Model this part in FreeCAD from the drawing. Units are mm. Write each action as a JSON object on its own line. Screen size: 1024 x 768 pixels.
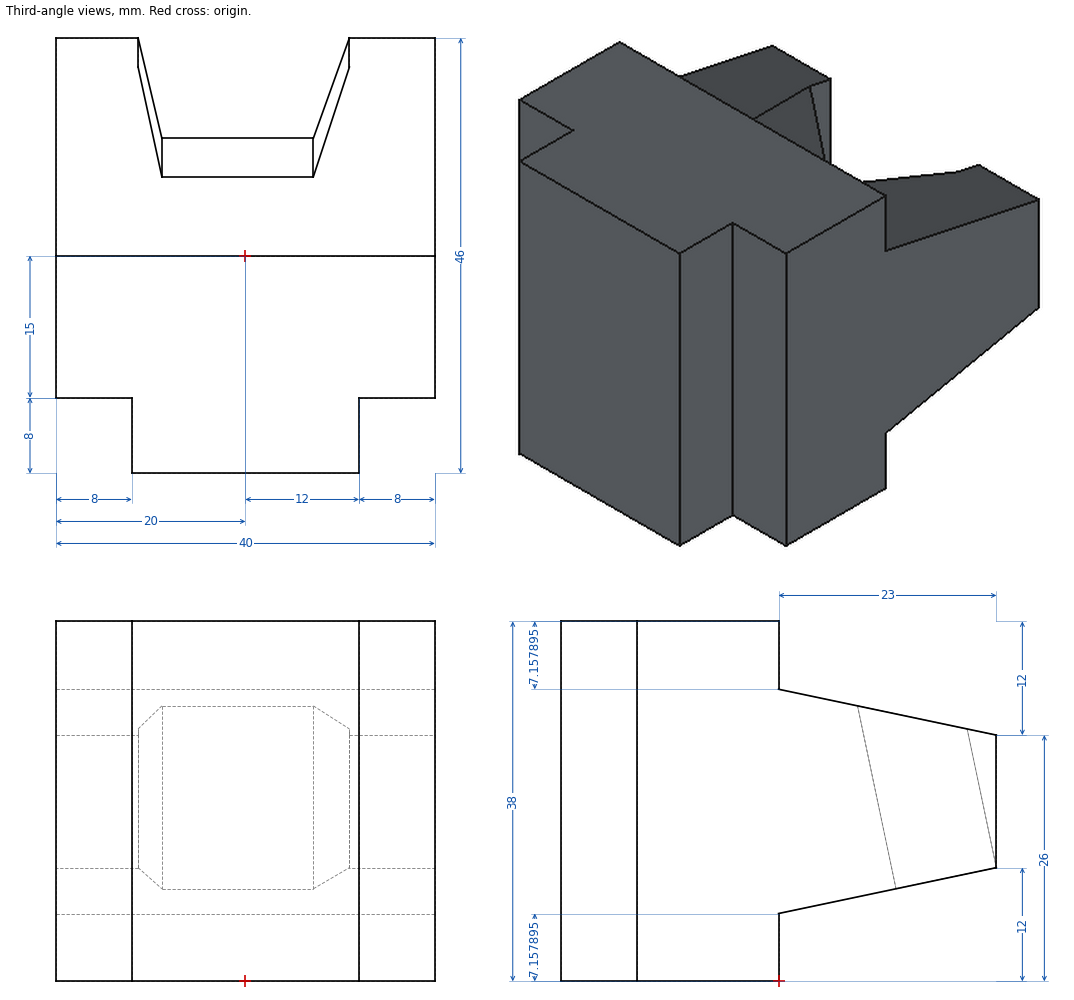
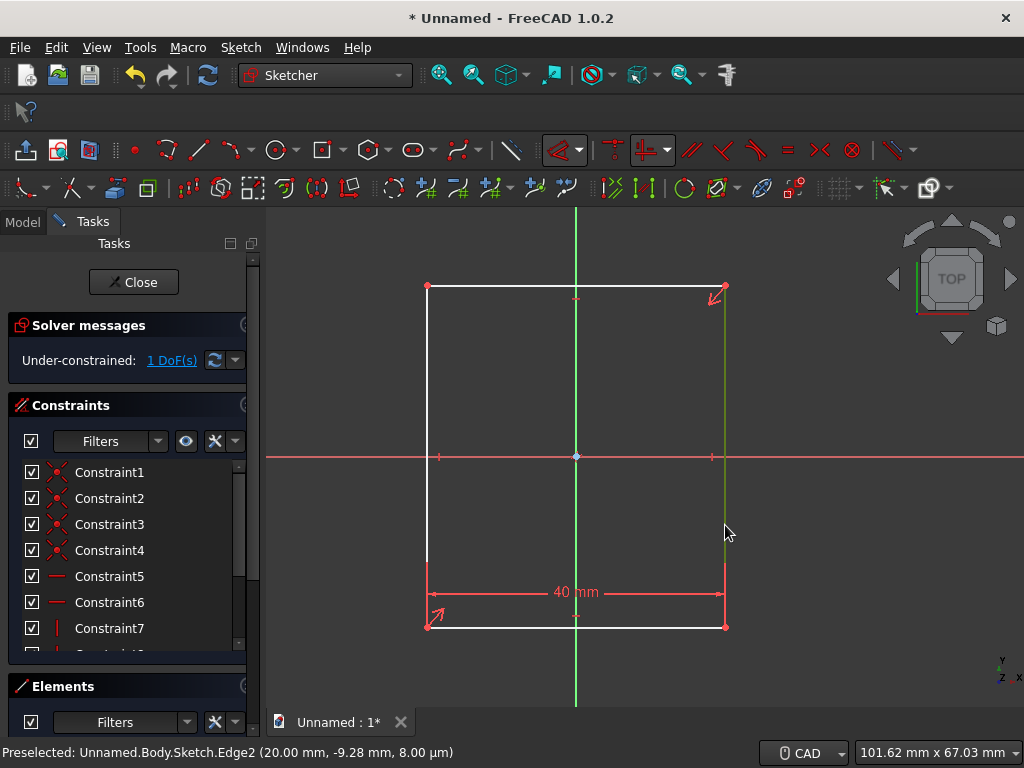
{"action": "left_click", "coordinate": [582, 150]}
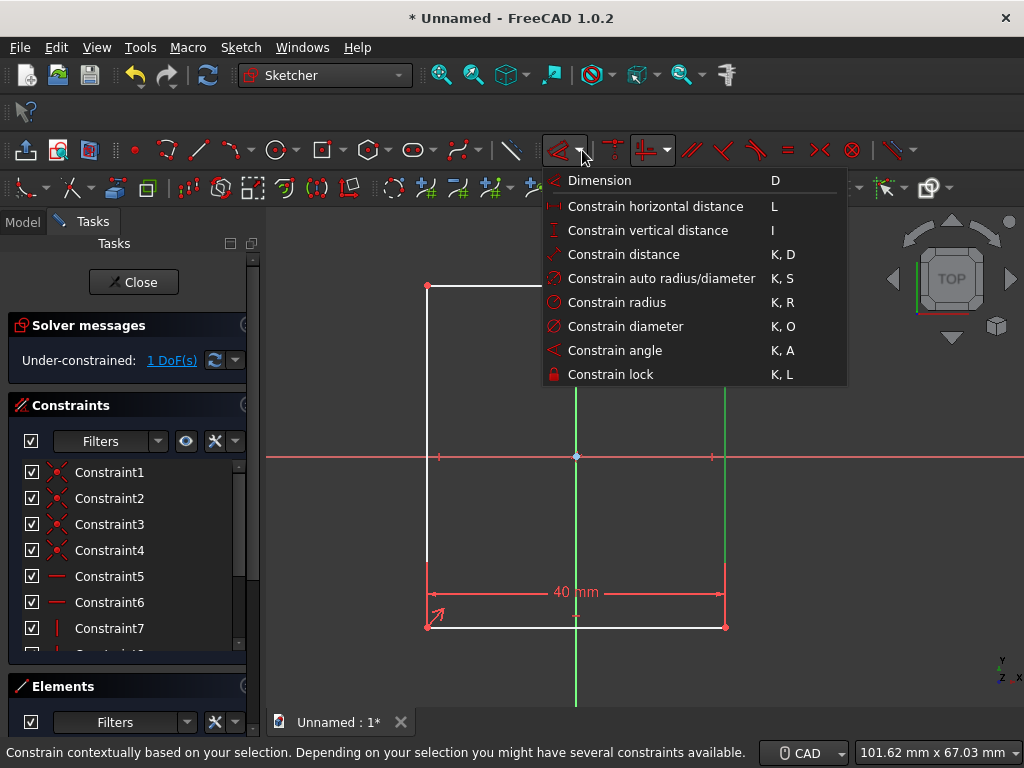
{"action": "left_click", "coordinate": [695, 230]}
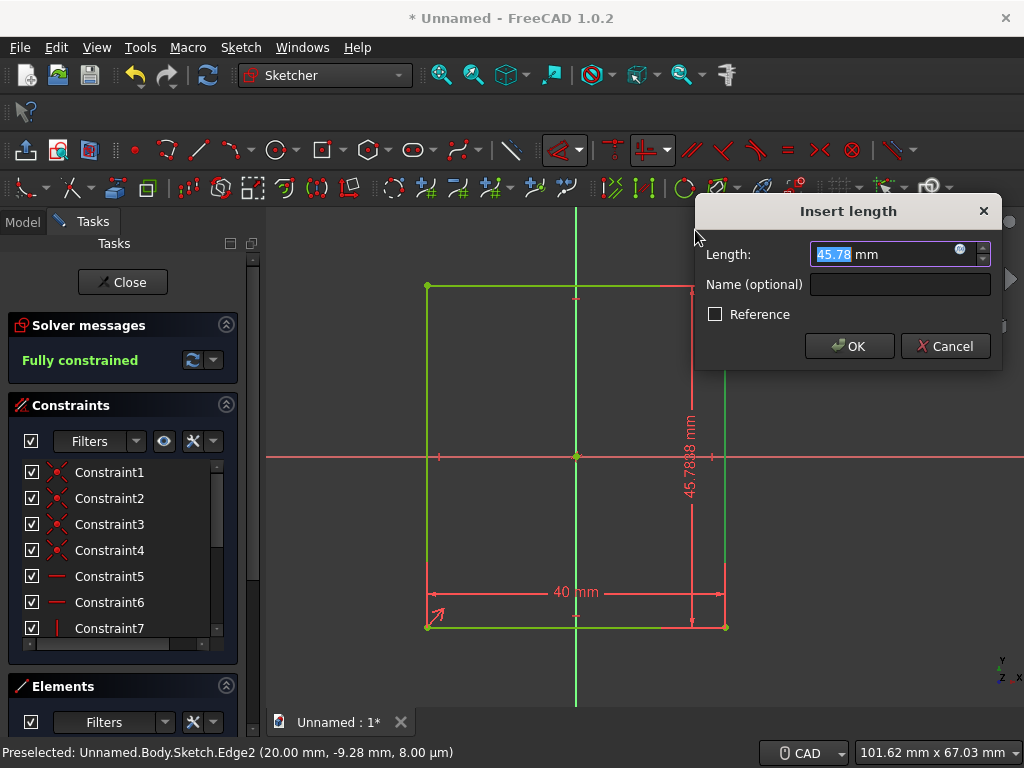
{"action": "type", "text": "46"}
{"action": "key", "text": "Return"}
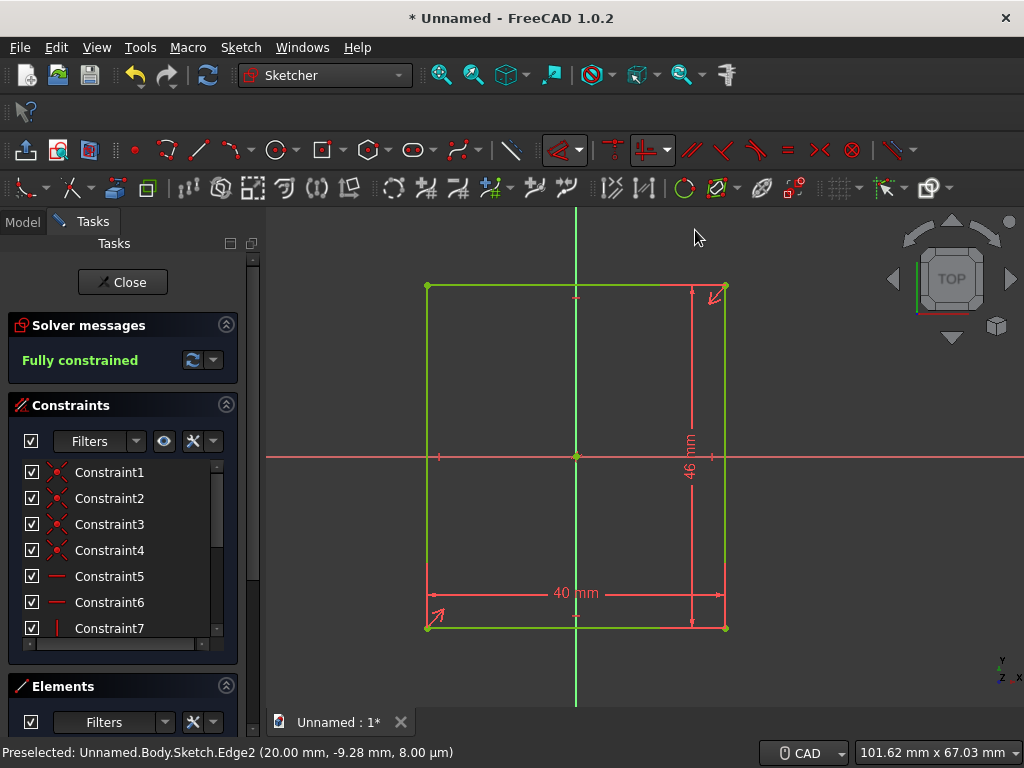
{"action": "left_click", "coordinate": [123, 282]}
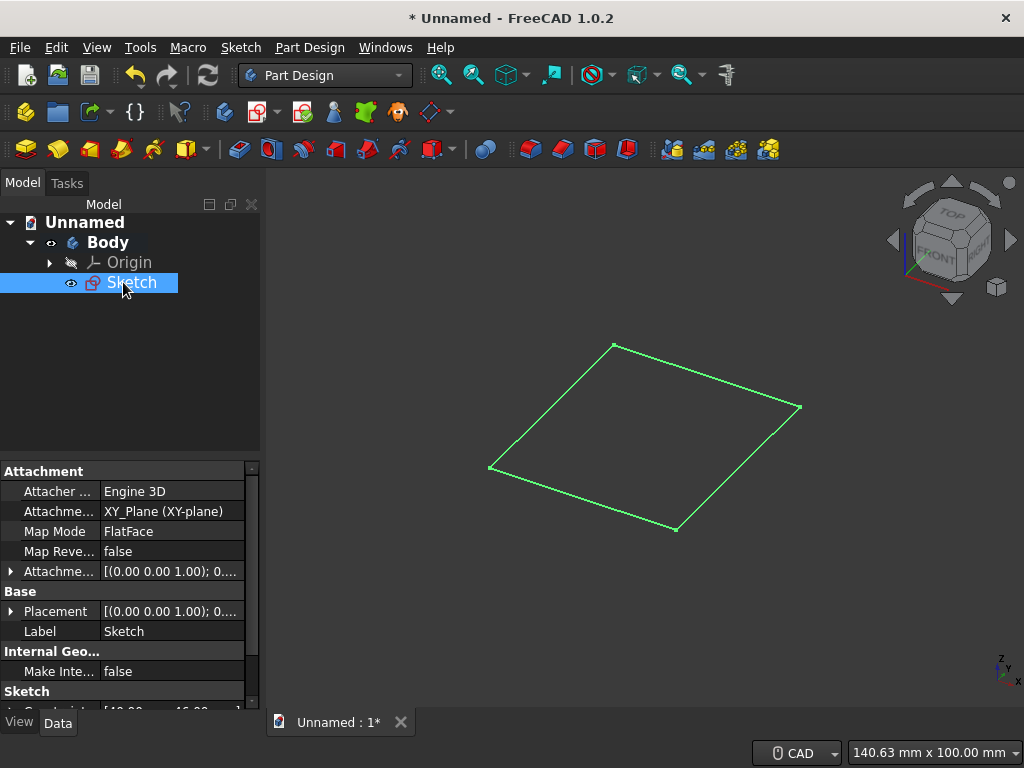
{"action": "left_click", "coordinate": [26, 150]}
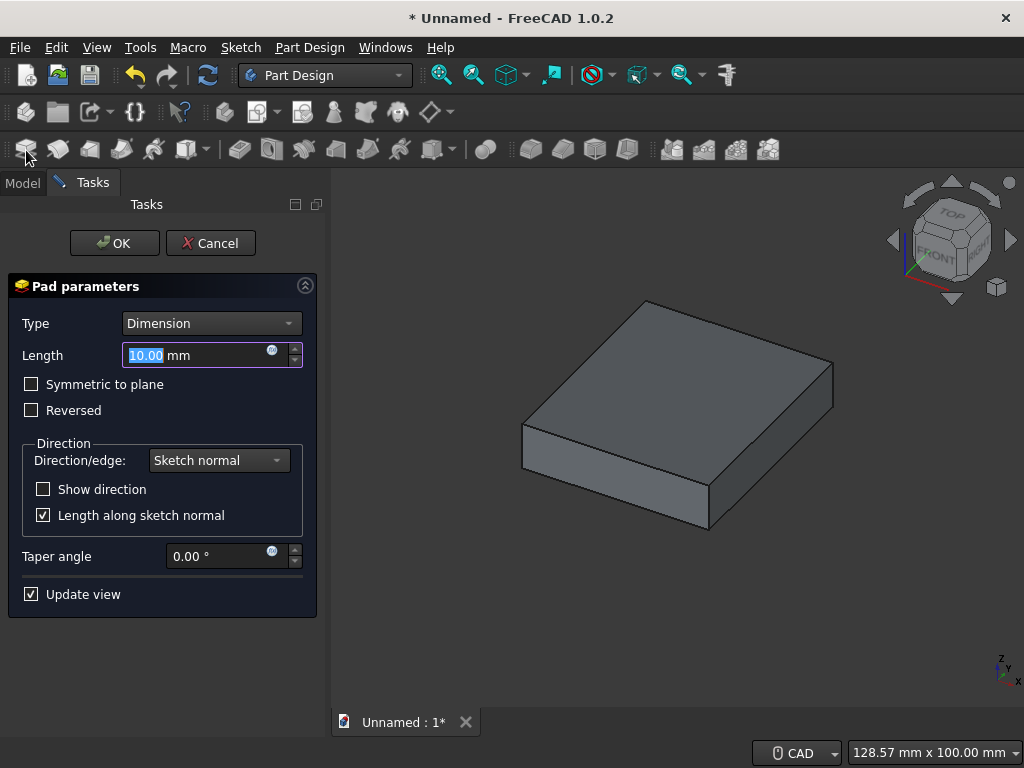
{"action": "type", "text": "38"}
{"action": "key", "text": "Tab"}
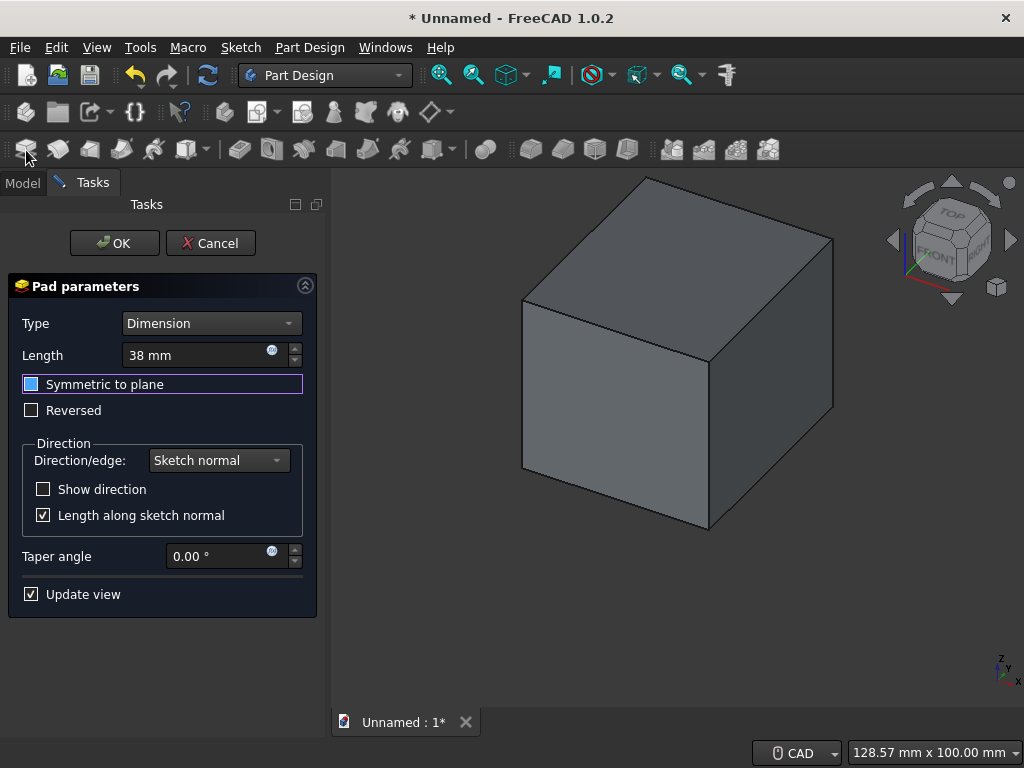
{"action": "left_click", "coordinate": [115, 243]}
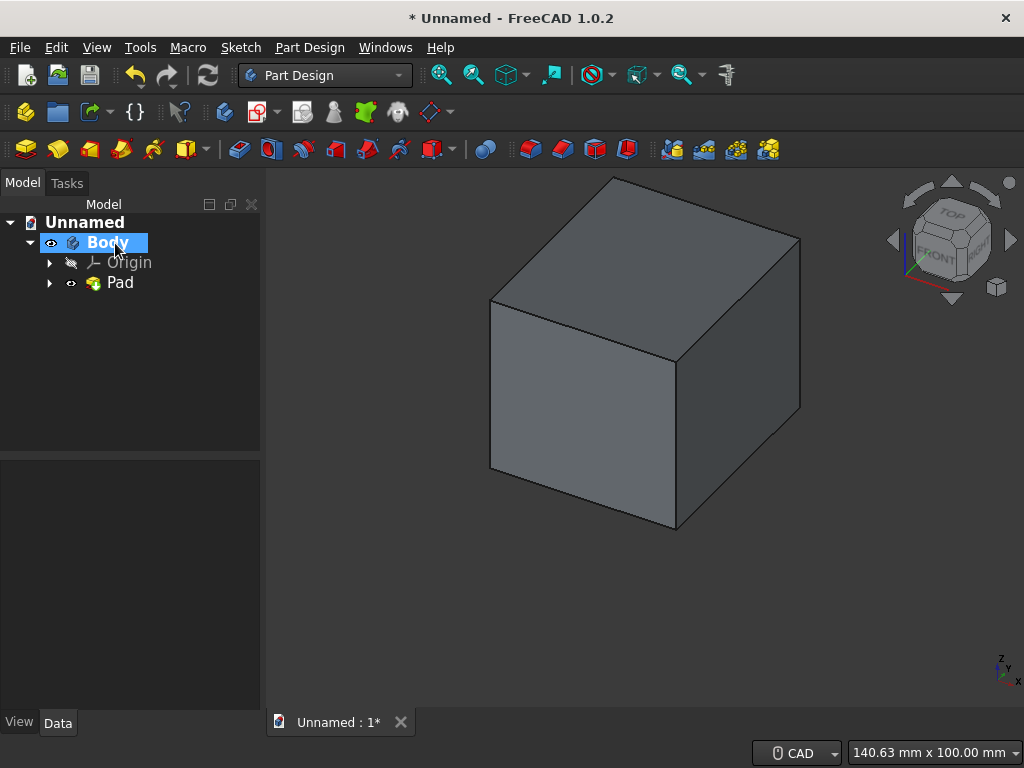
{"action": "left_click", "coordinate": [645, 269]}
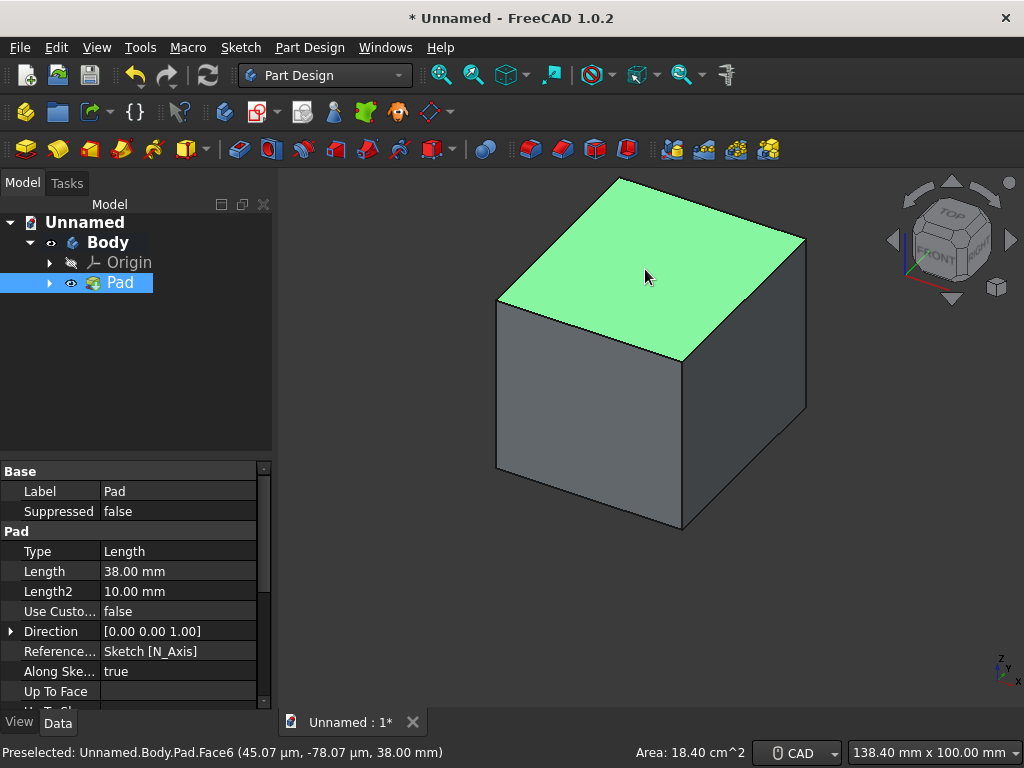
{"action": "left_click", "coordinate": [258, 112]}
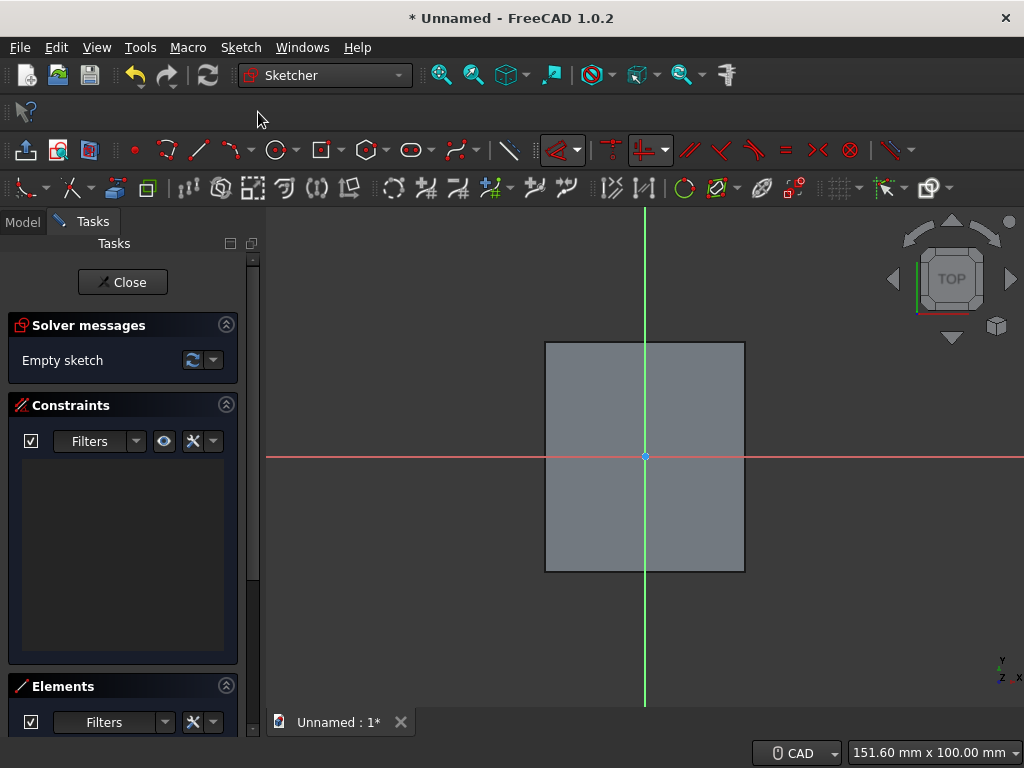
{"action": "scroll", "coordinate": [563, 567], "scroll_direction": "up", "scroll_amount": 10}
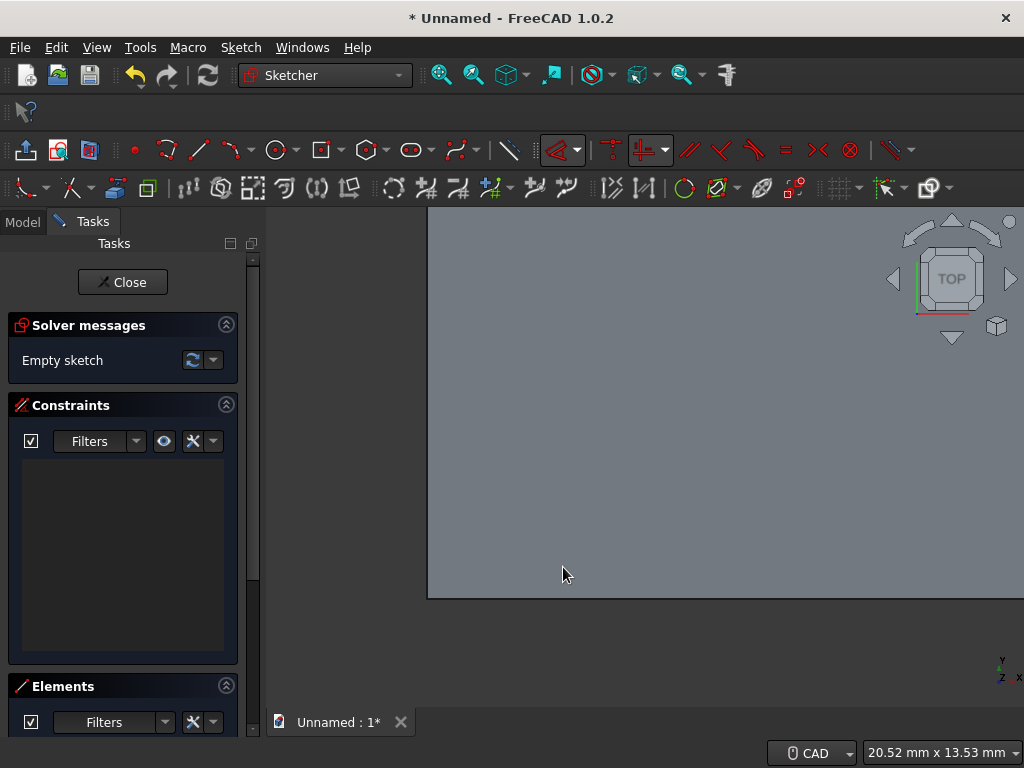
{"action": "left_click", "coordinate": [344, 150]}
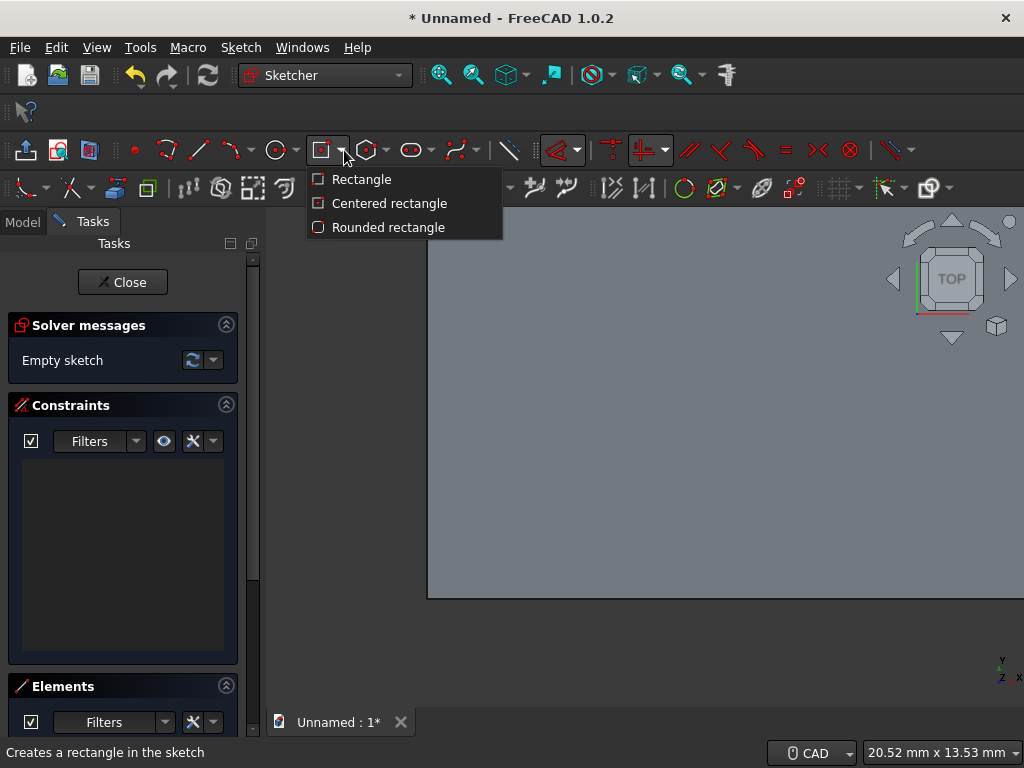
{"action": "left_click", "coordinate": [404, 179]}